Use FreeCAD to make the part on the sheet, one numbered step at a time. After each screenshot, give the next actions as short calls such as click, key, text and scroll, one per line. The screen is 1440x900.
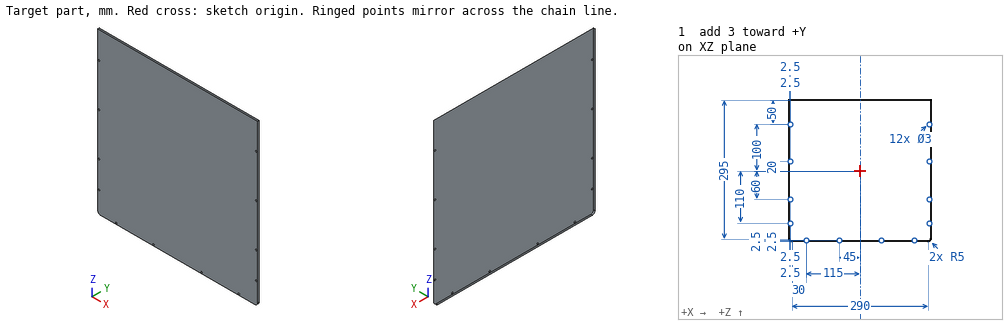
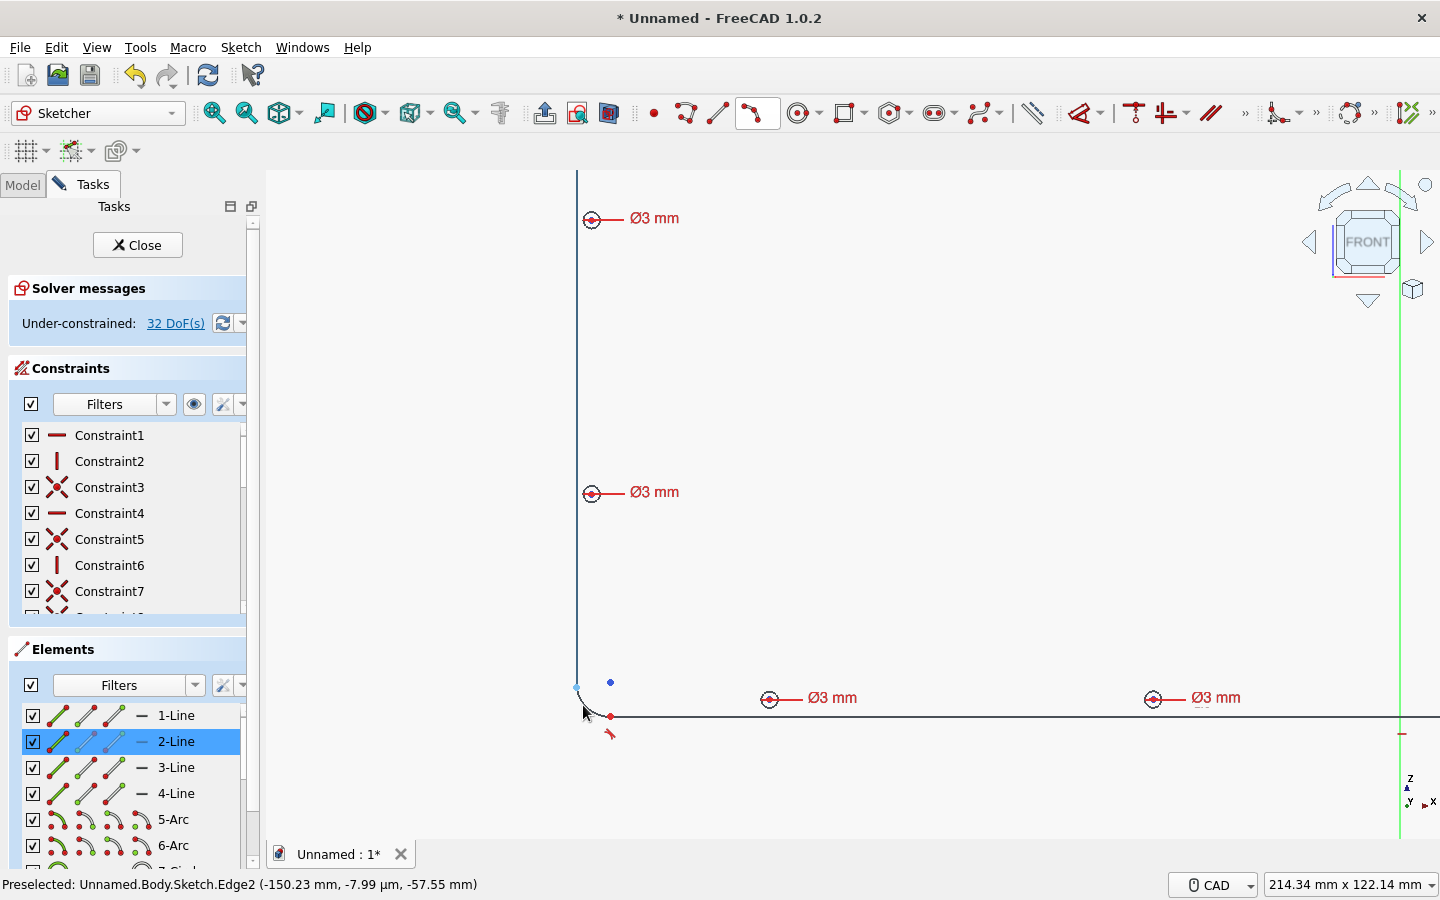
click(582, 701)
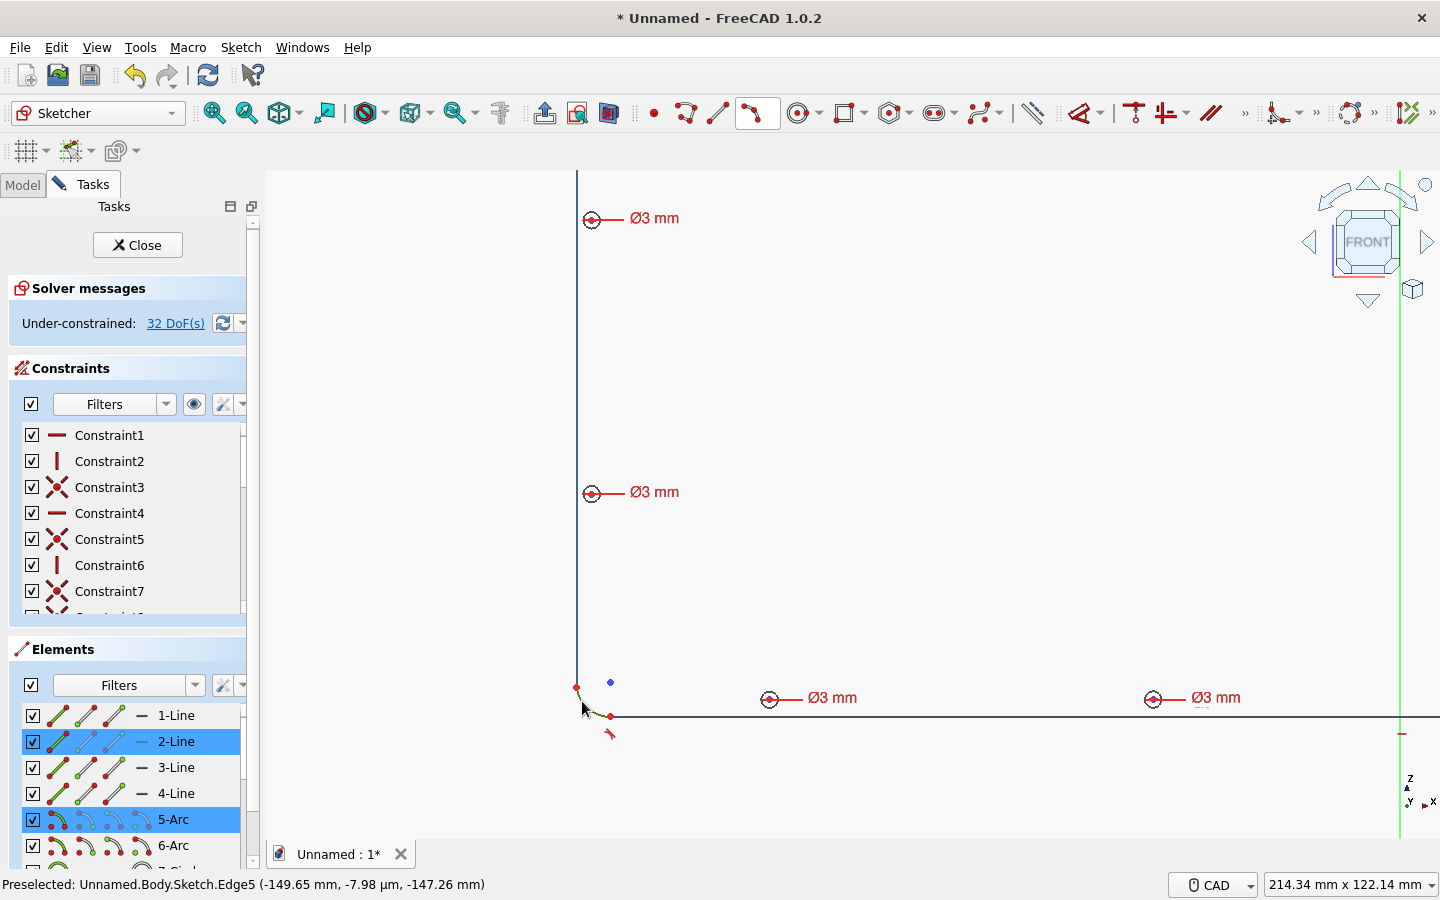
key(t)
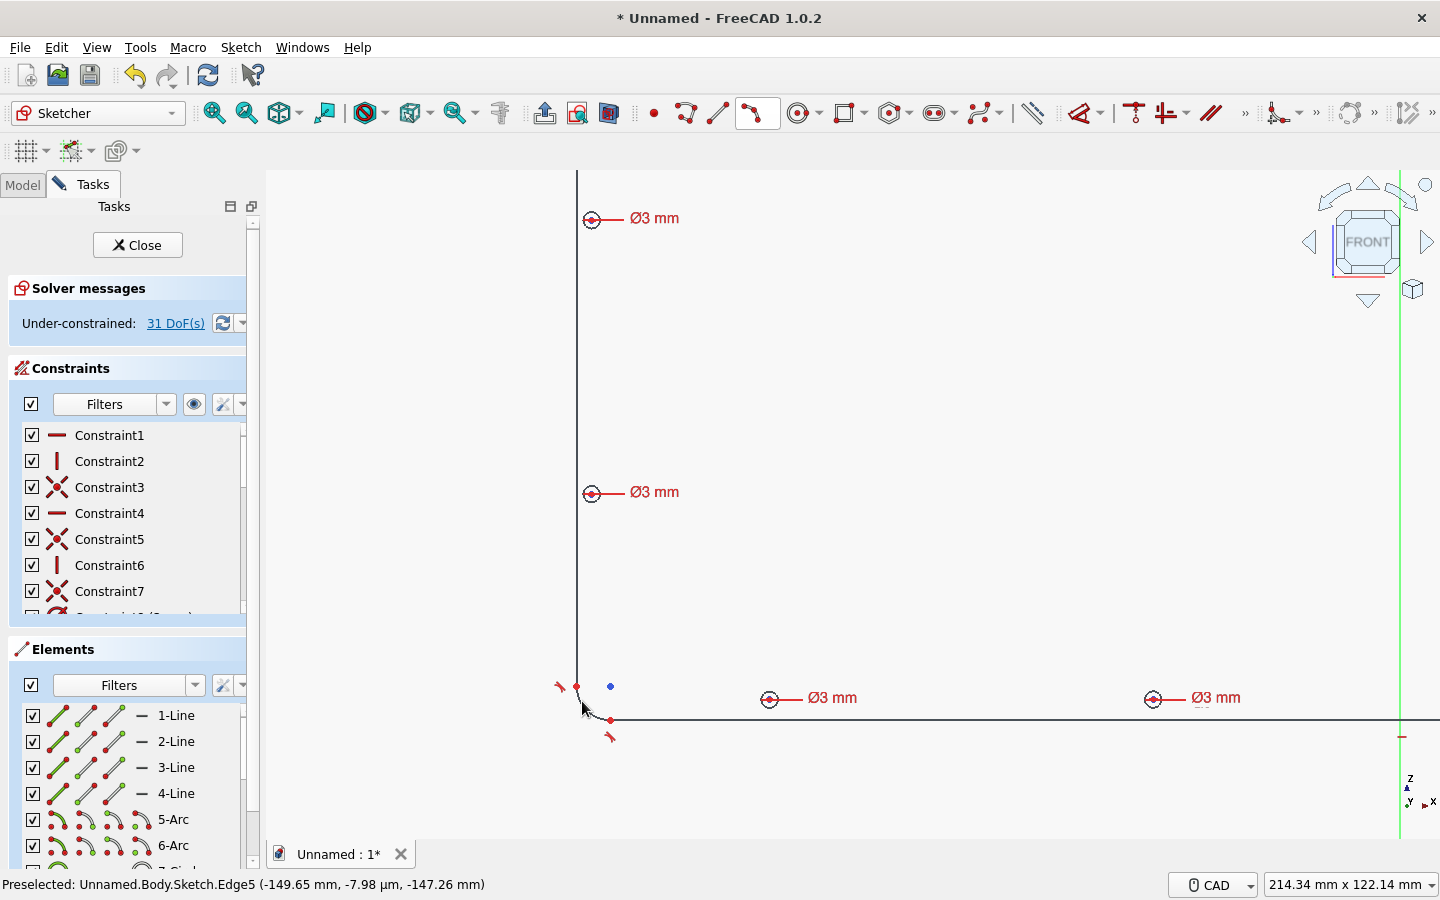
scroll(583, 705, down, 7)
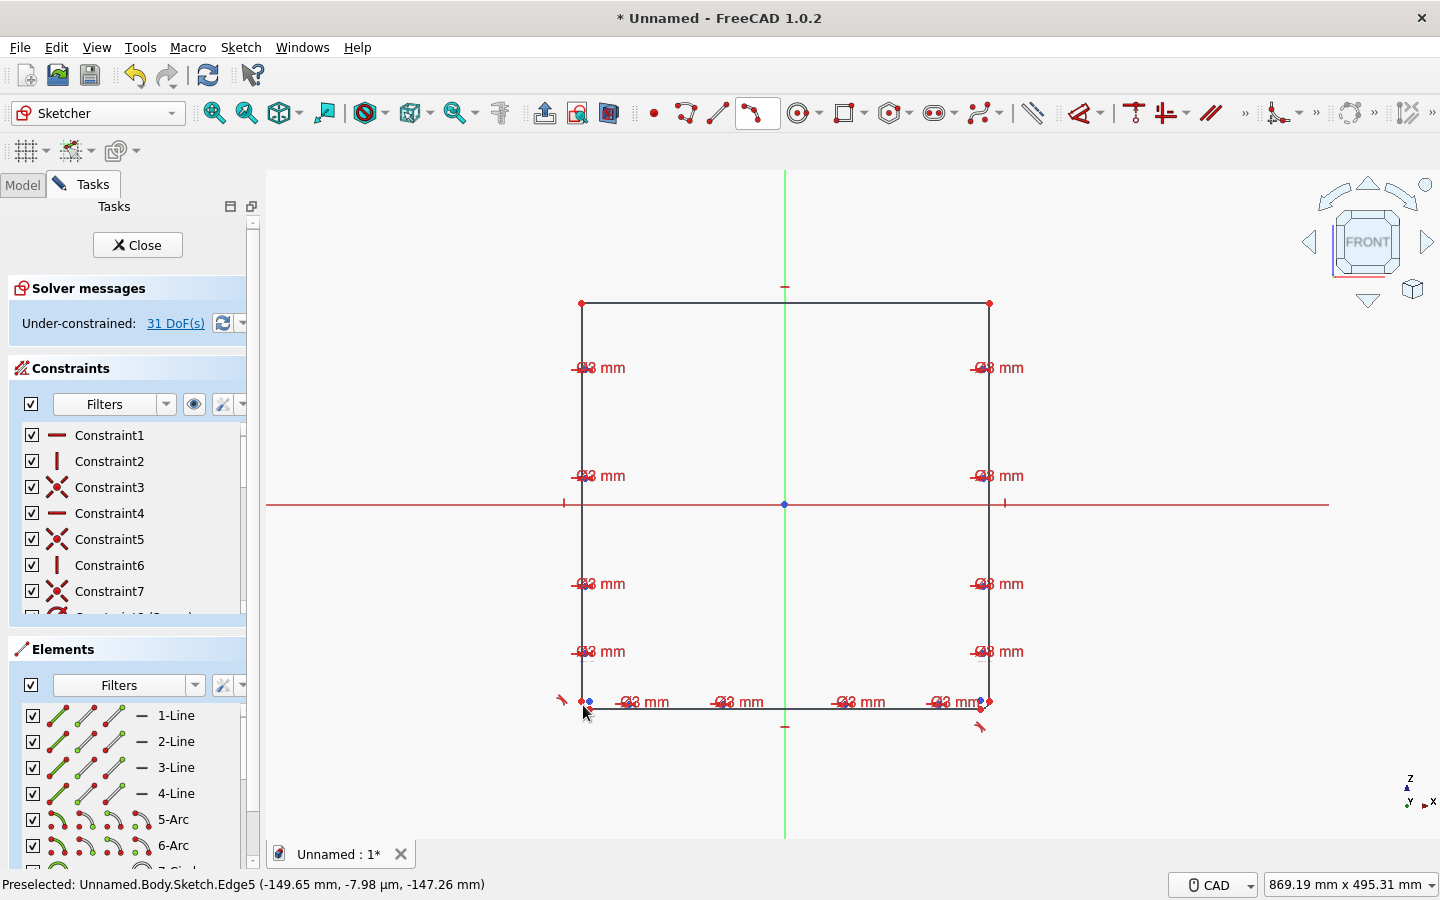
click(989, 423)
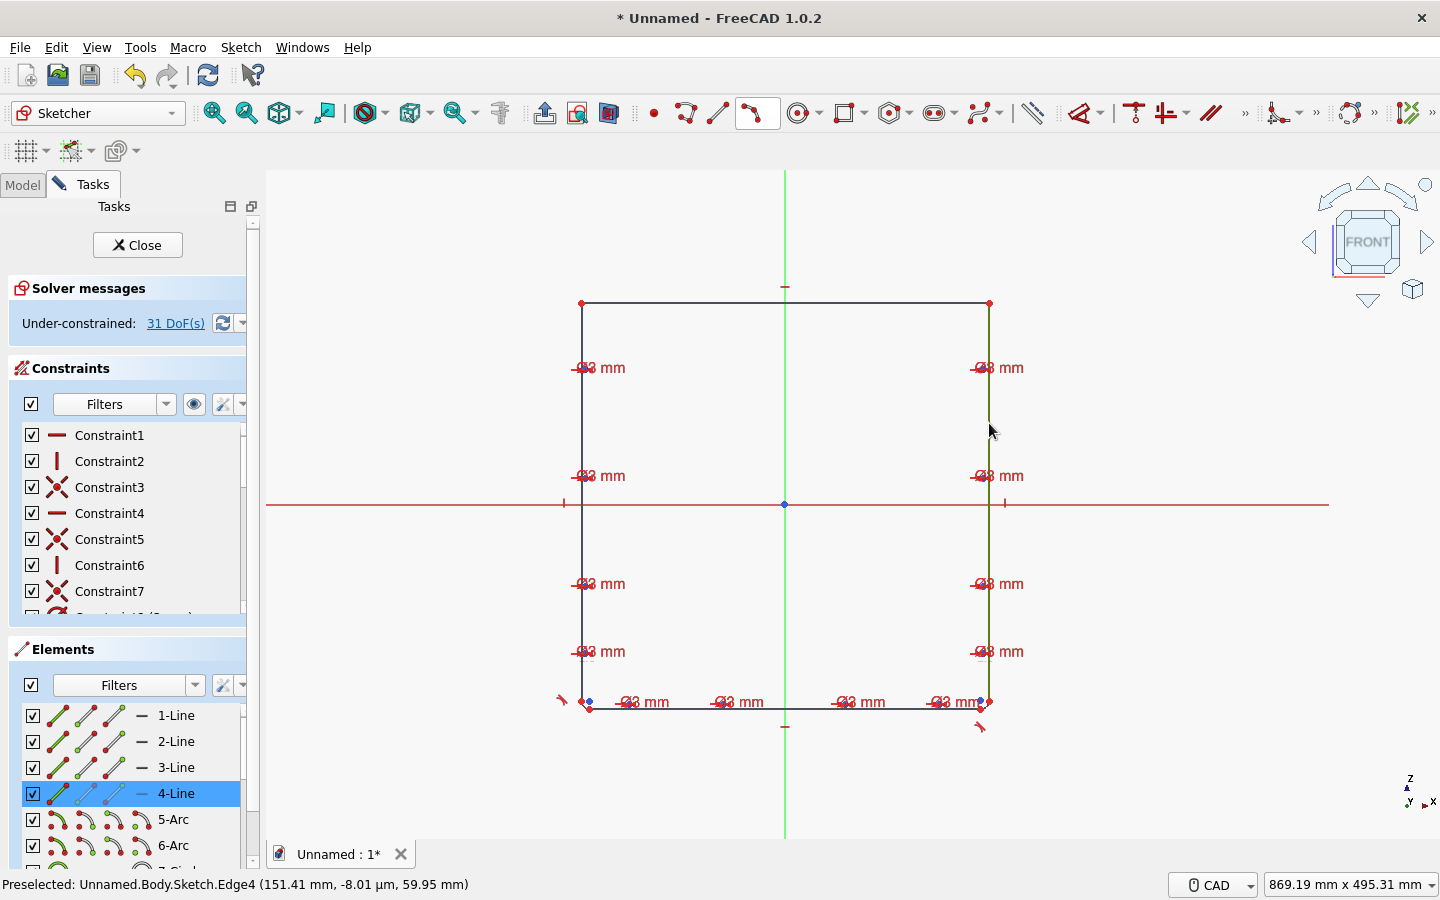
scroll(986, 707, up, 4)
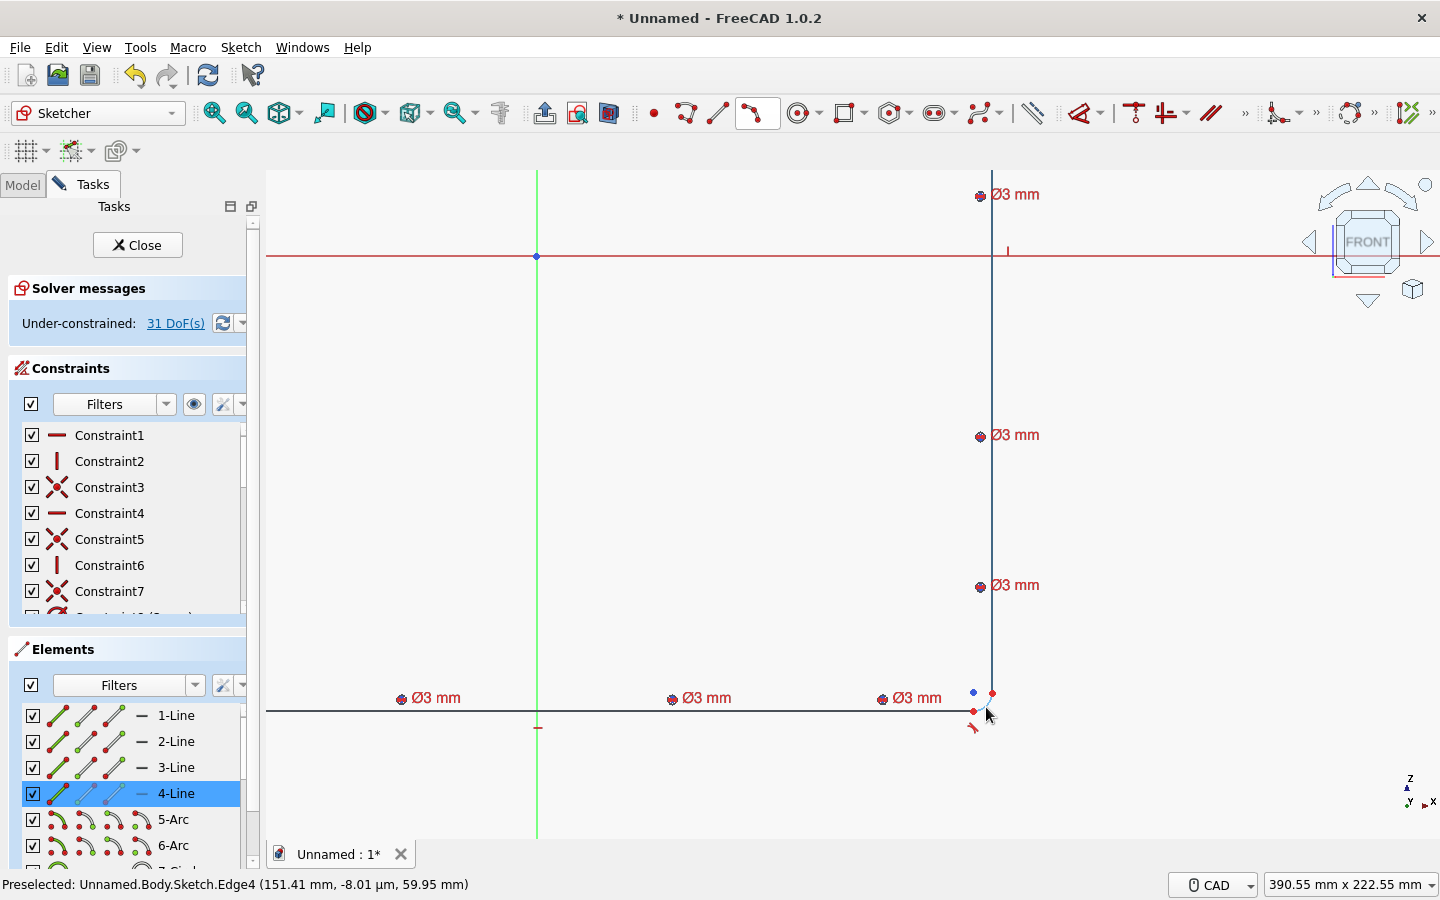
click(986, 706)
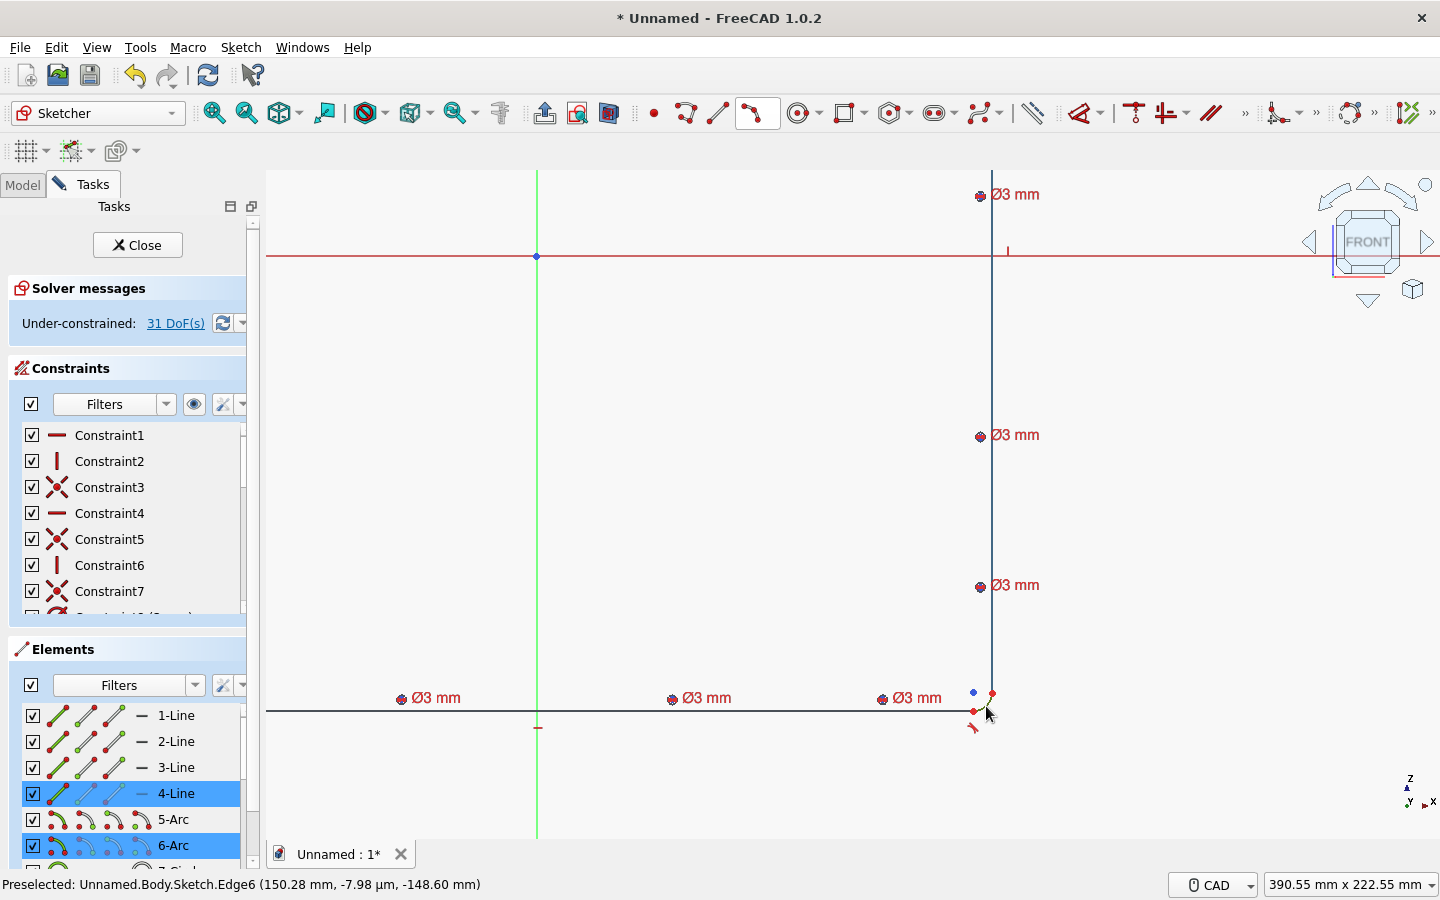
key(t)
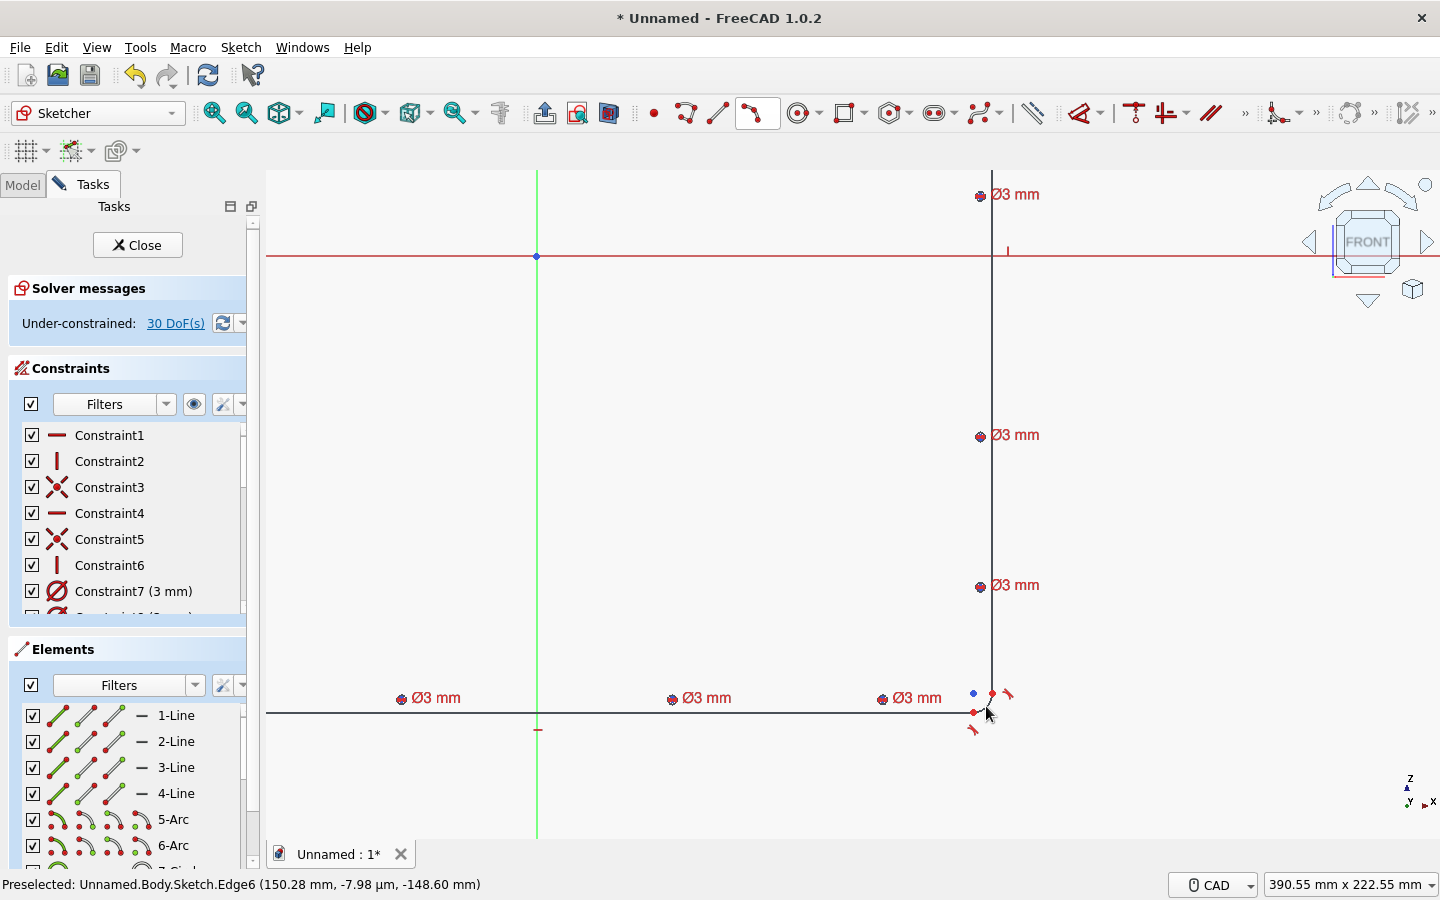
scroll(986, 707, down, 4)